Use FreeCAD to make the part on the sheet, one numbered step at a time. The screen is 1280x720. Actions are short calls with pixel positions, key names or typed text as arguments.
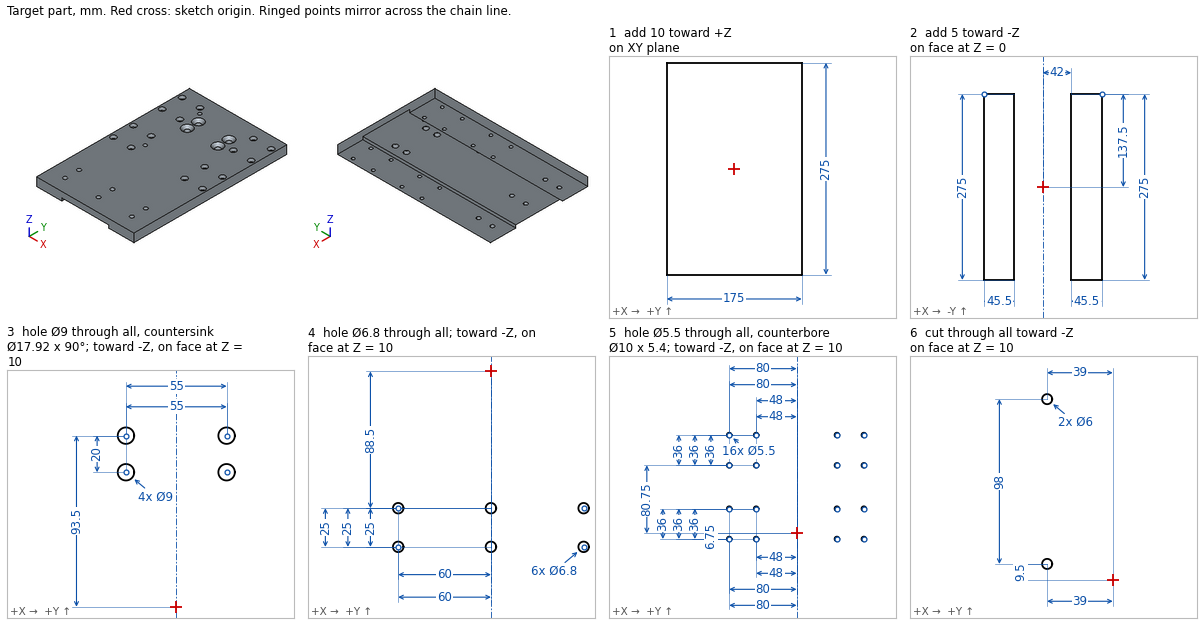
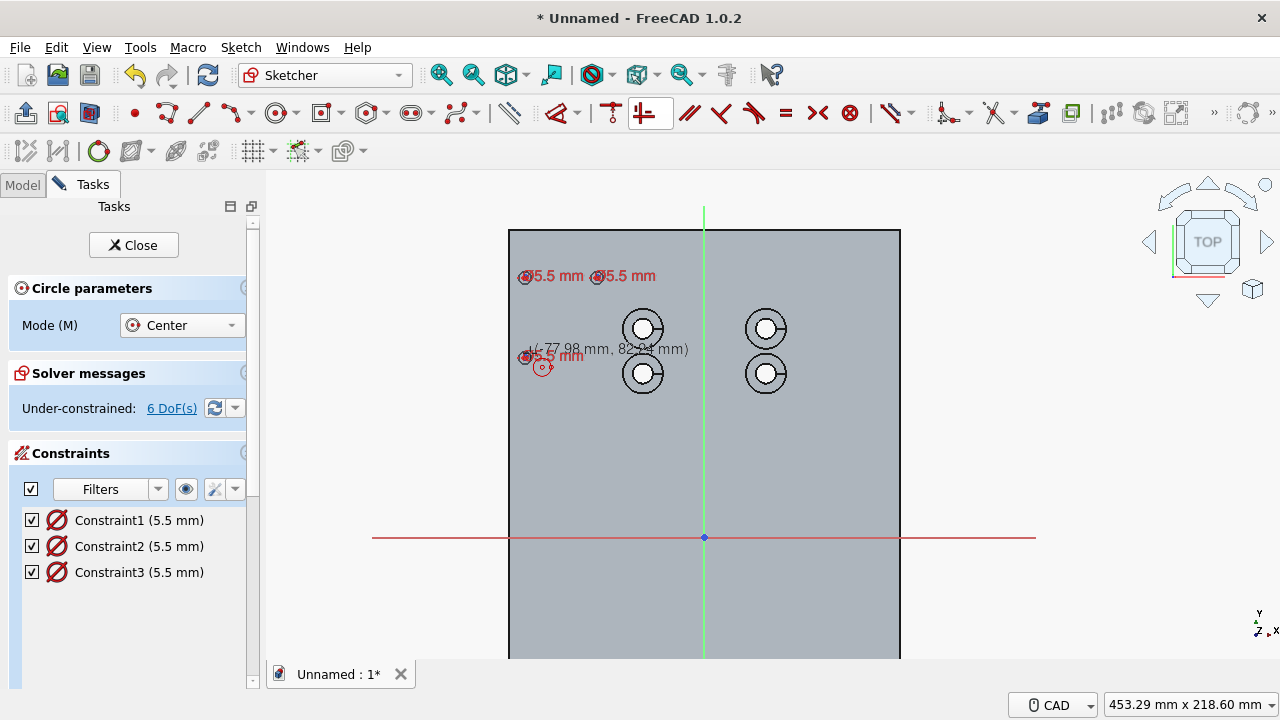
scroll(597, 357, up, 7)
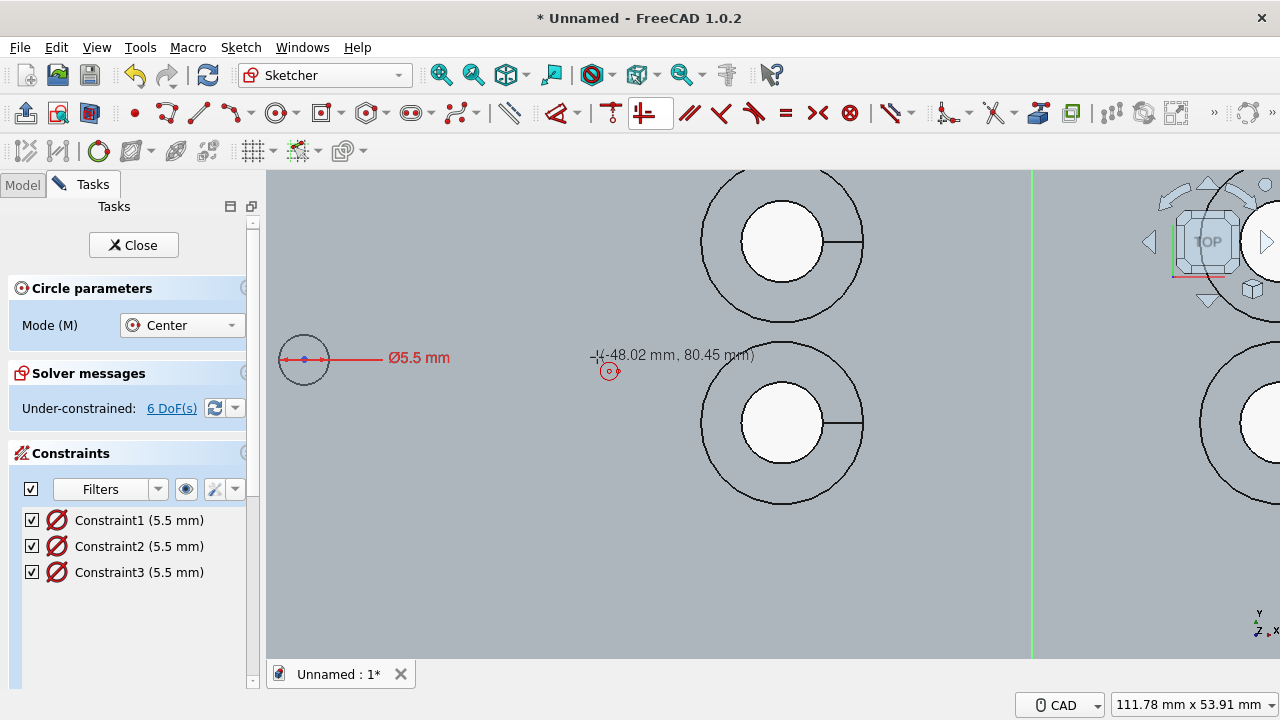
scroll(597, 357, down, 7)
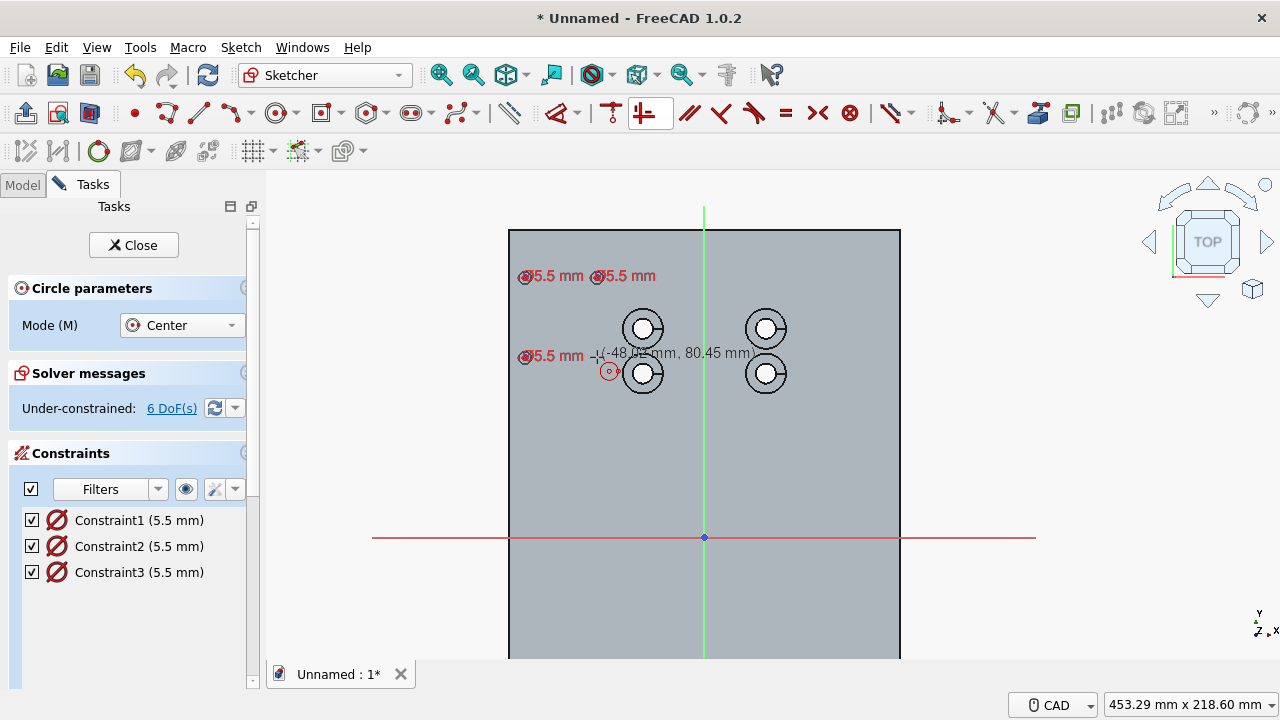
click(597, 357)
move(601, 353)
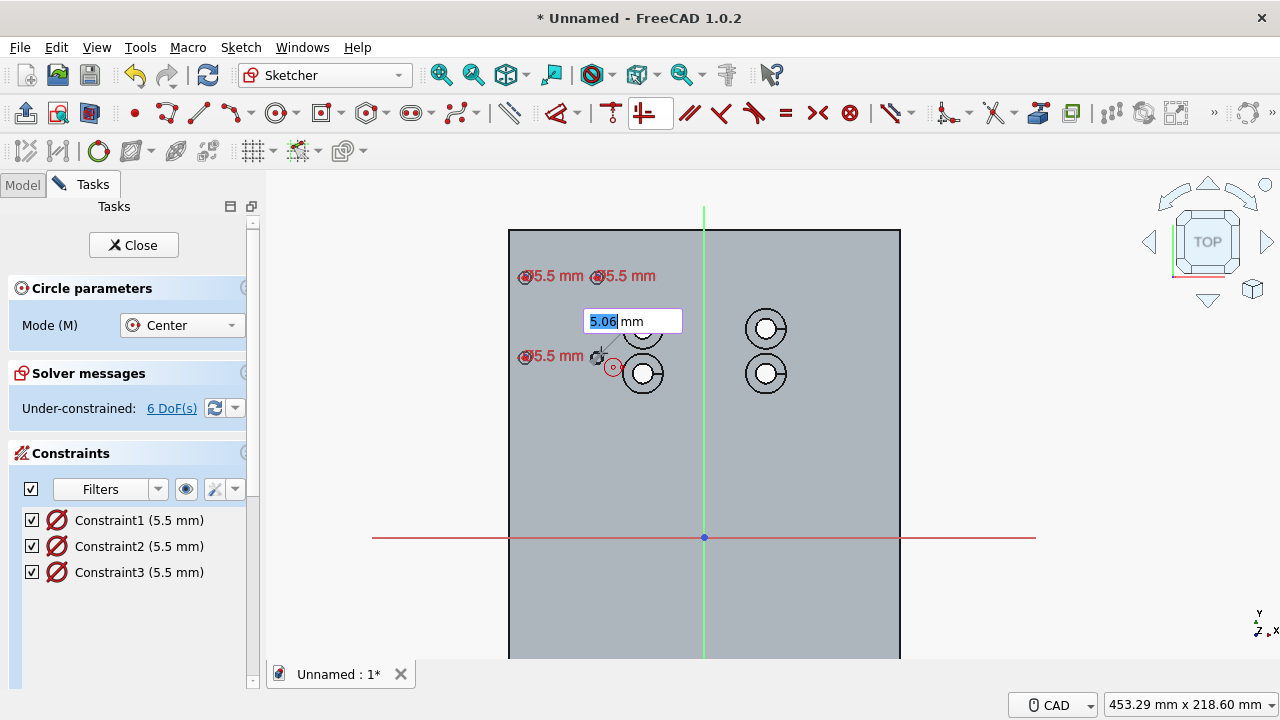
text(5.5)
key(Return)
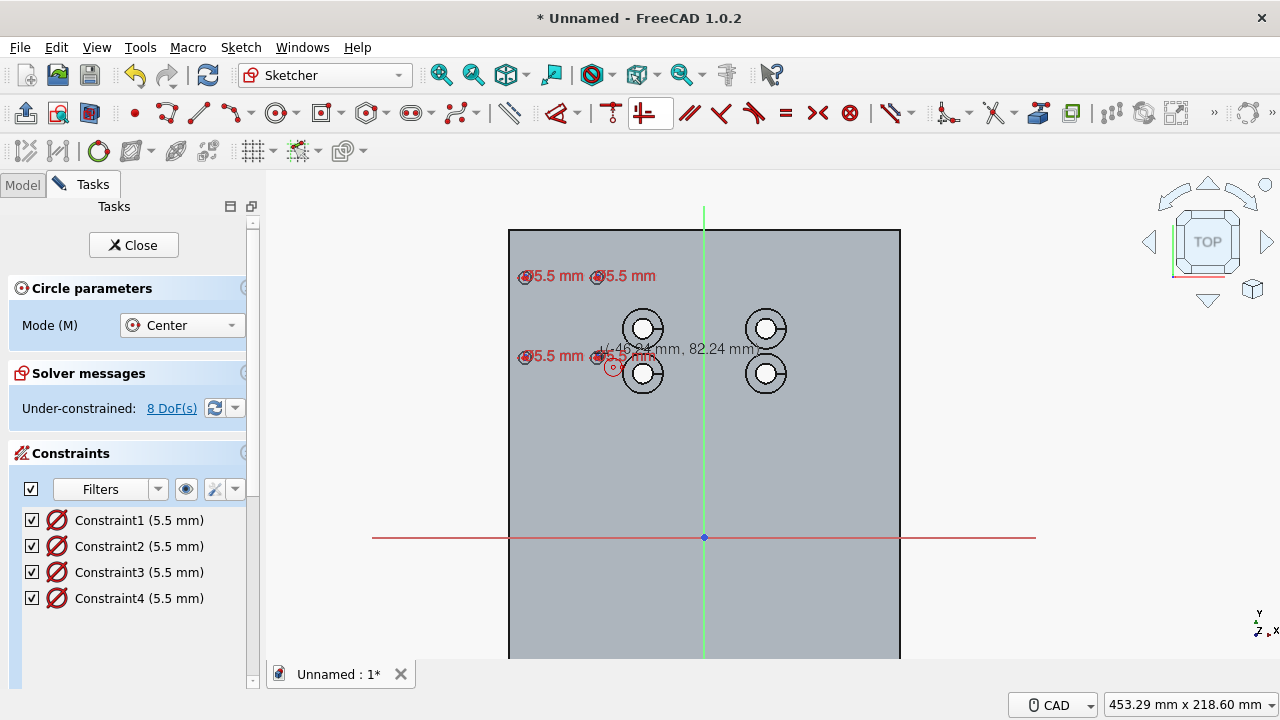
scroll(525, 473, up, 7)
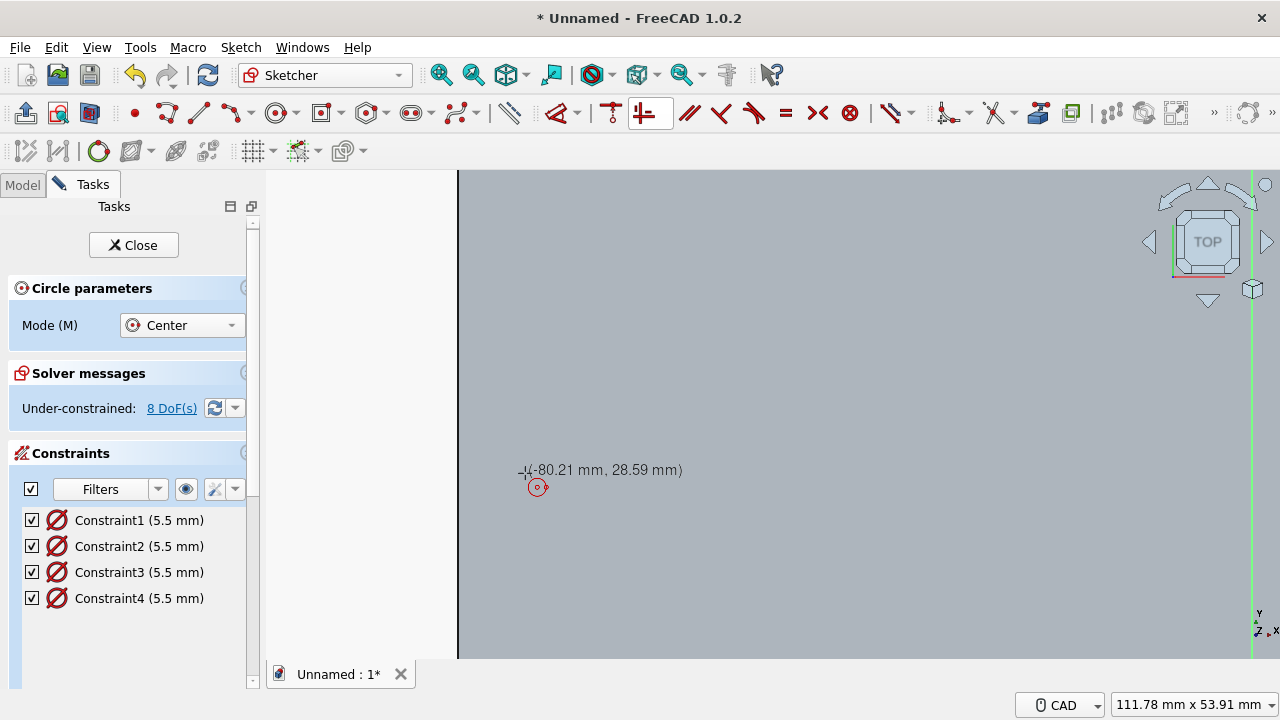
scroll(525, 473, down, 7)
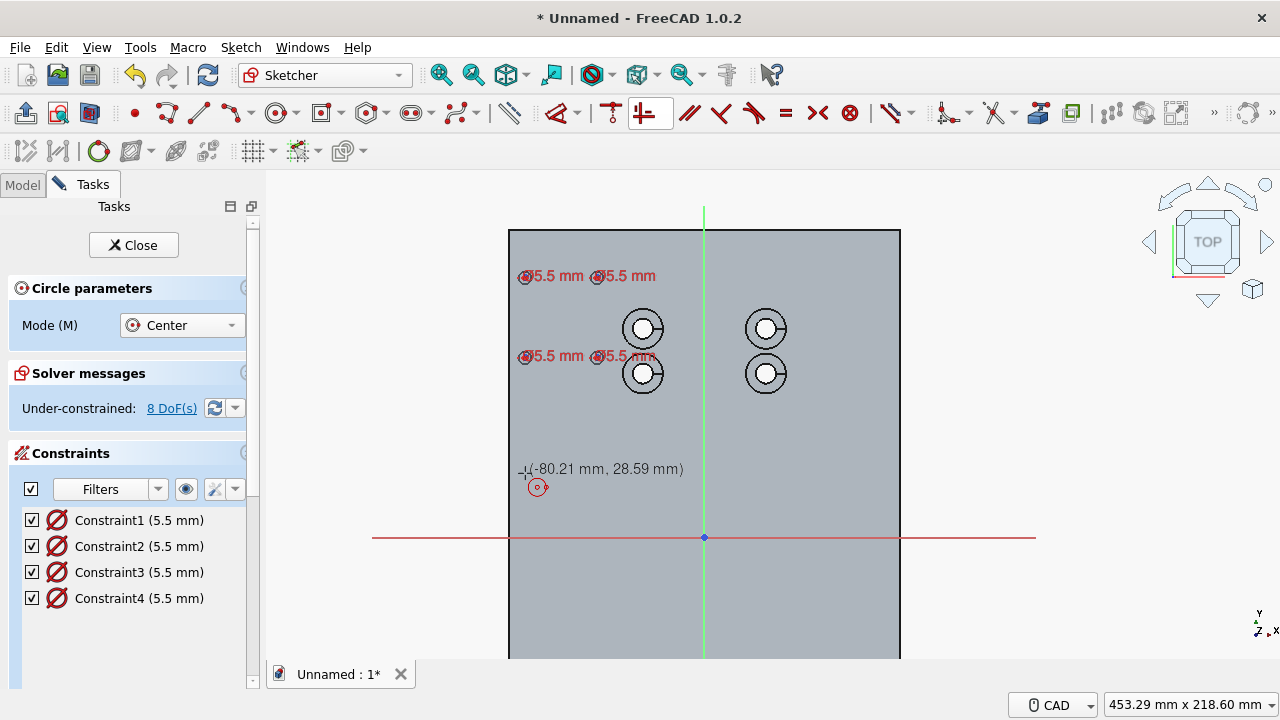
click(525, 473)
move(530, 468)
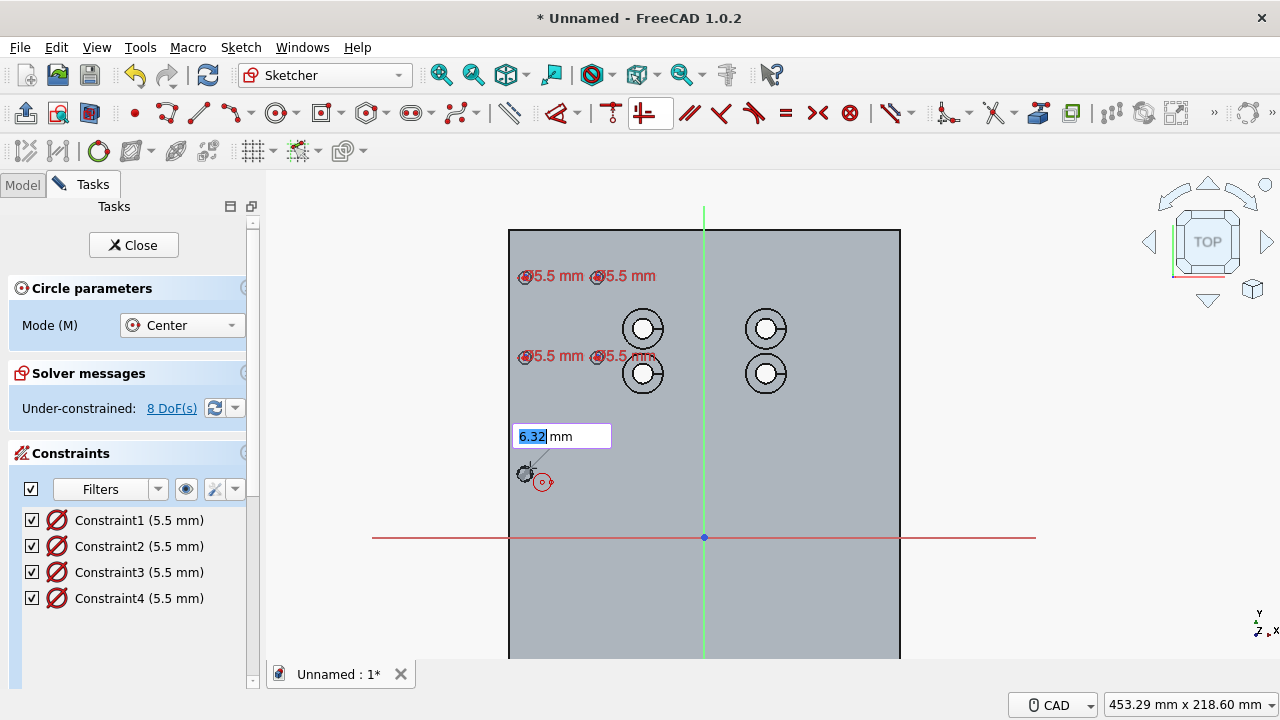
text(5.5)
key(Return)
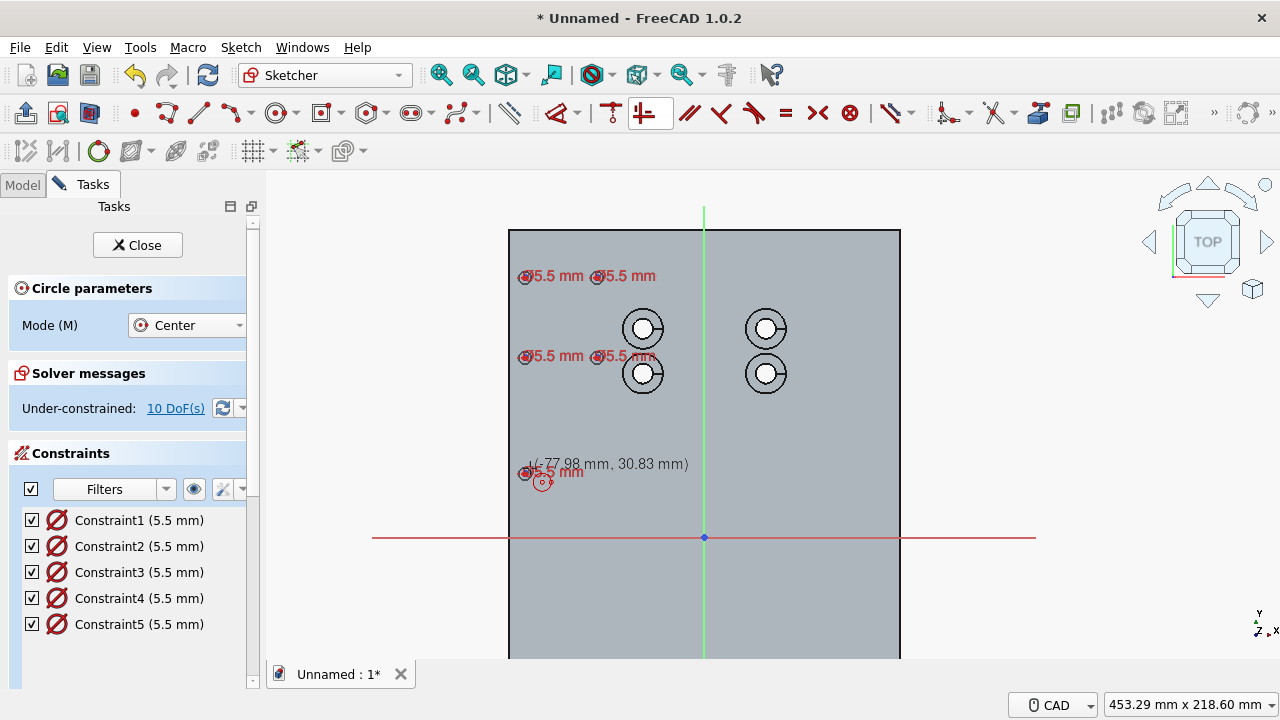
scroll(597, 473, up, 7)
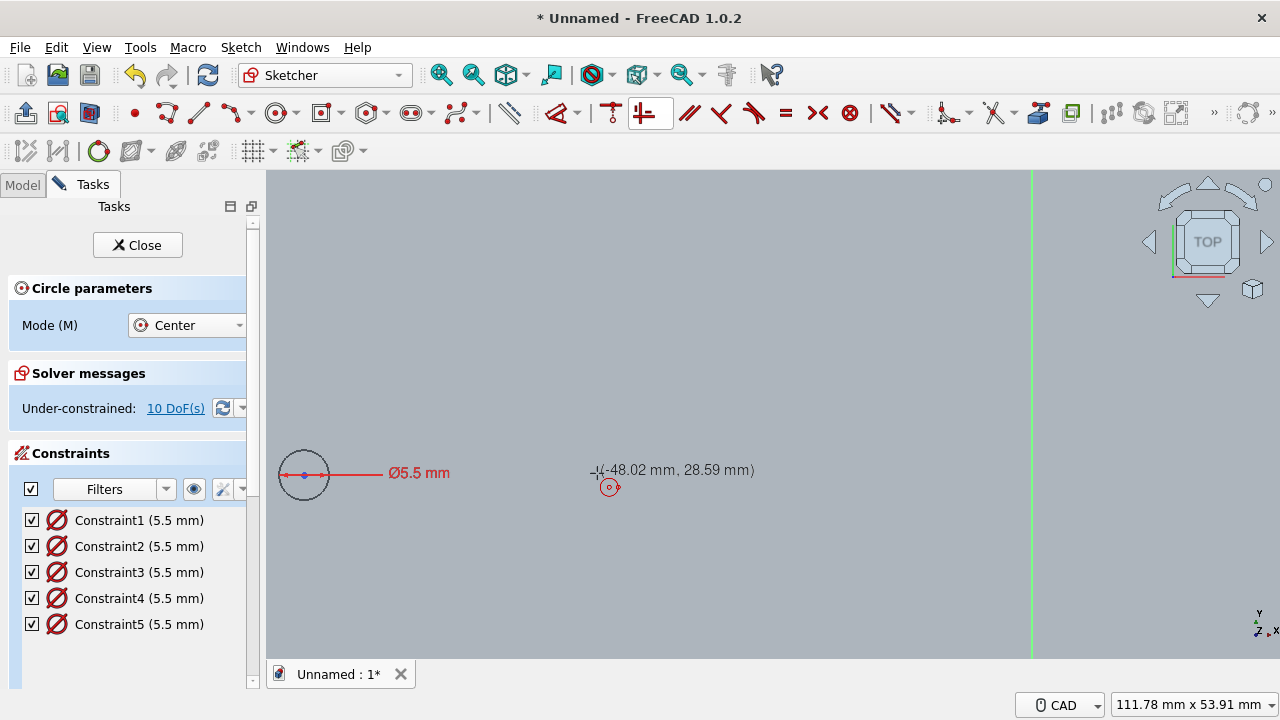
scroll(597, 473, down, 7)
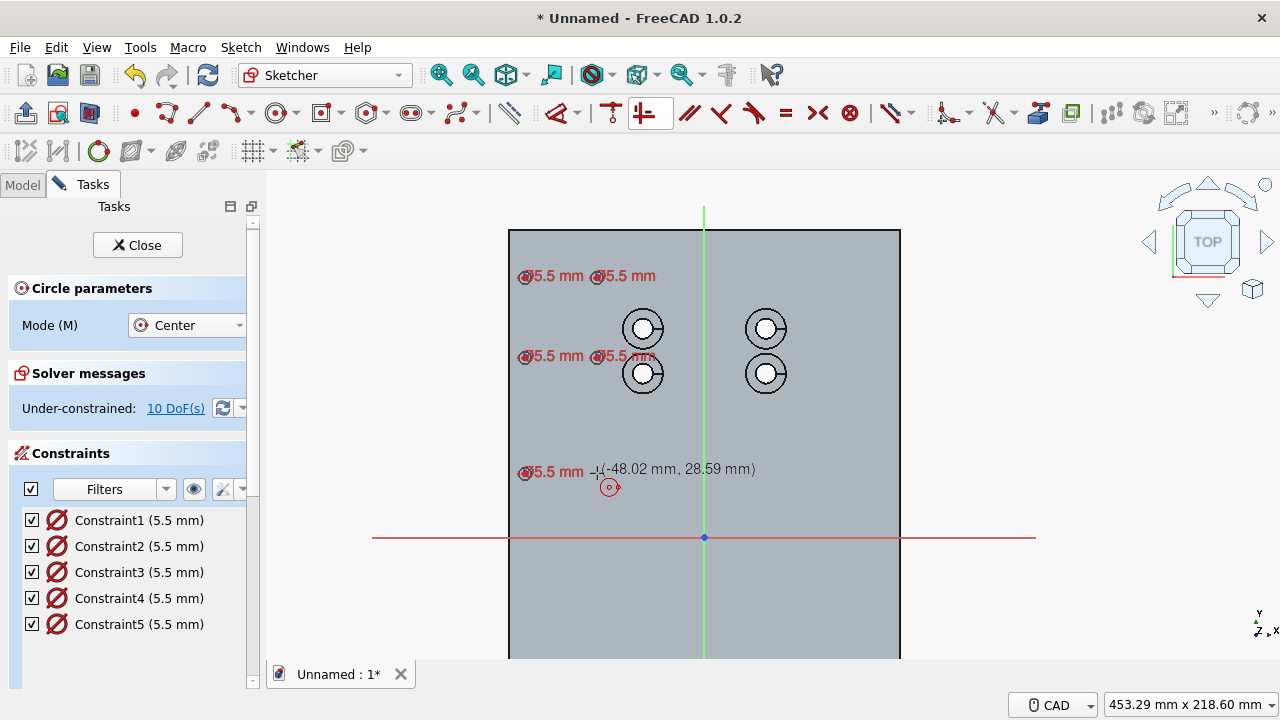
click(597, 473)
move(601, 468)